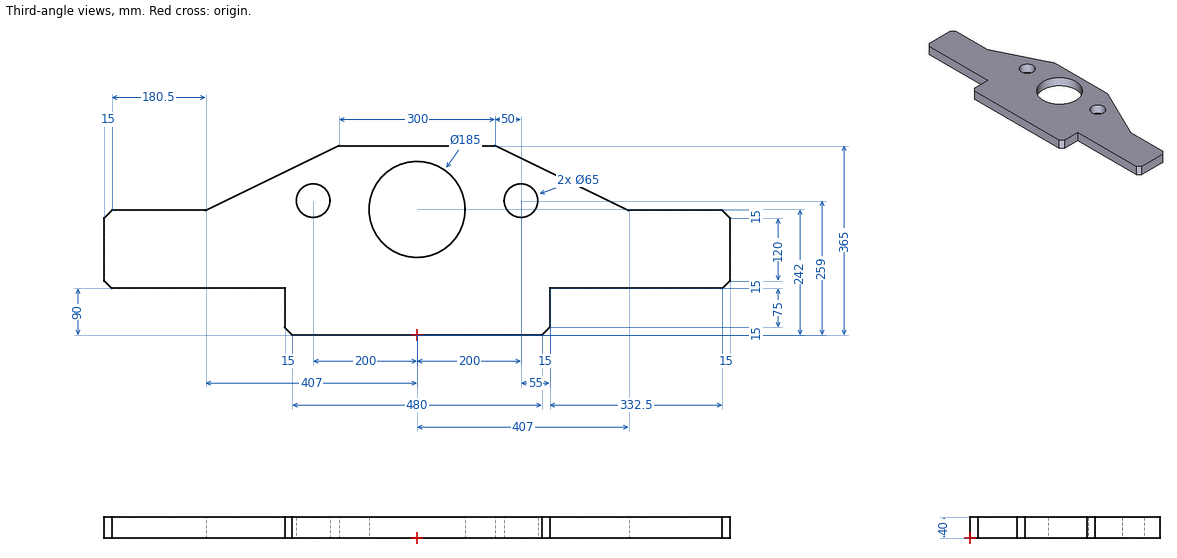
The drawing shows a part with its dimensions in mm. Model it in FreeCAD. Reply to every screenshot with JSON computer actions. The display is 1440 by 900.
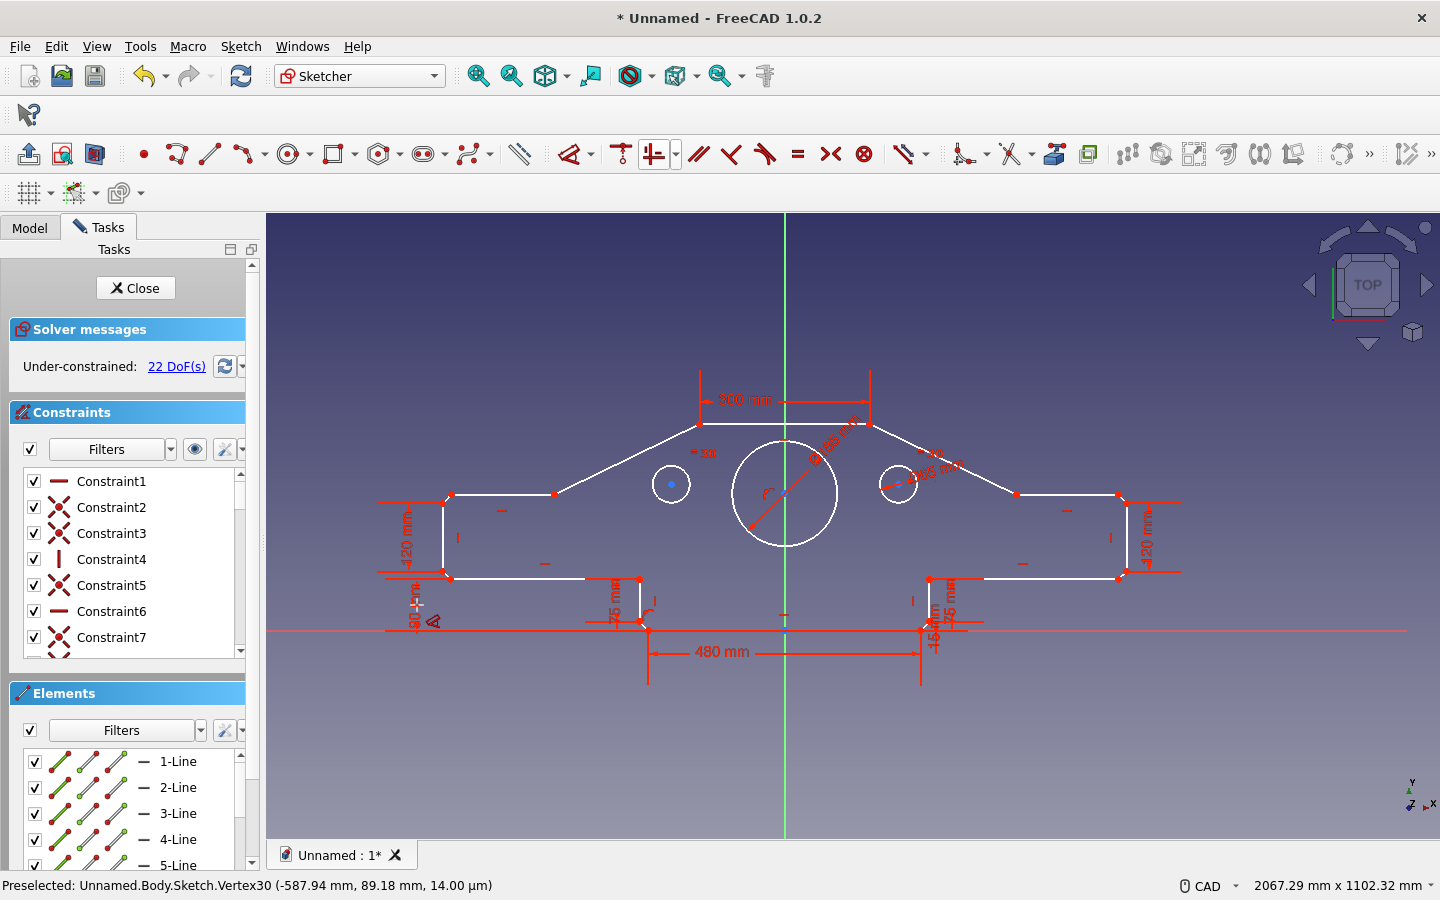
{"action": "scroll", "coordinate": [926, 625], "scroll_direction": "up", "scroll_amount": 8}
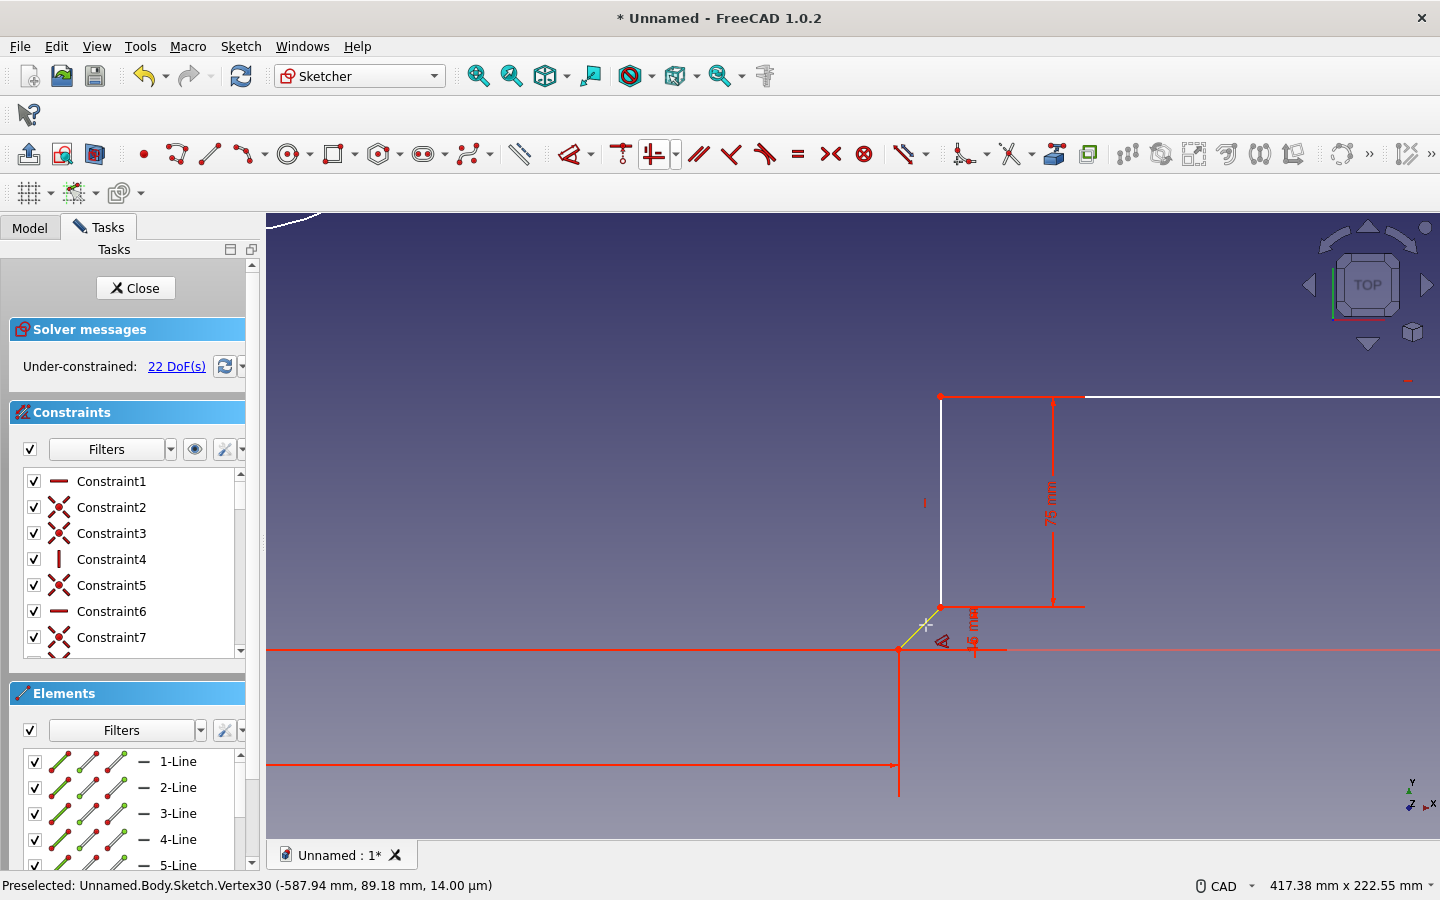
{"action": "left_click", "coordinate": [924, 624]}
{"action": "left_click", "coordinate": [920, 684]}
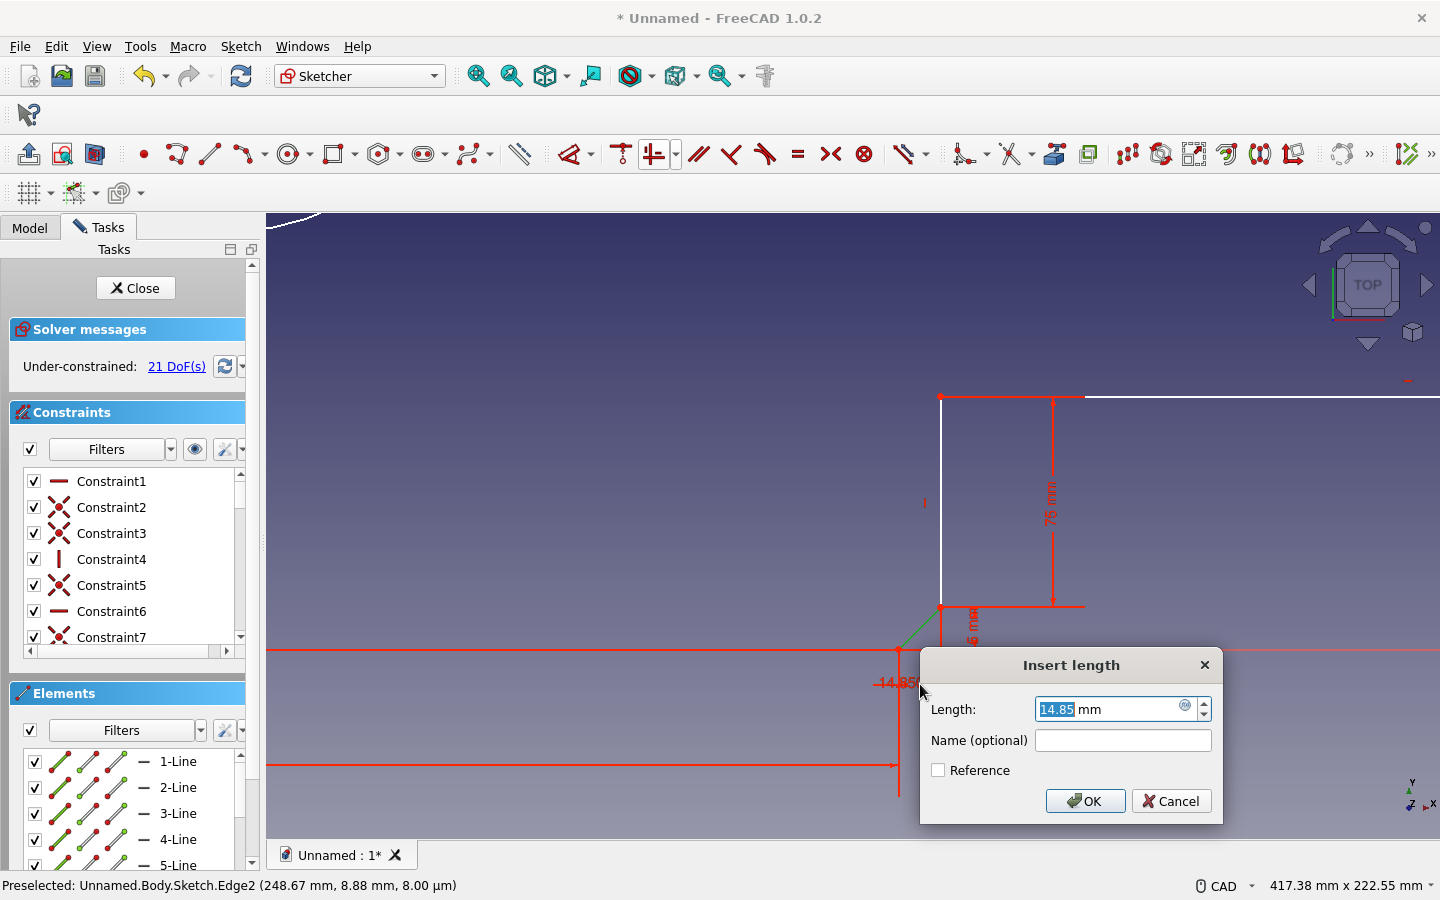
{"action": "type", "text": "15"}
{"action": "key", "text": "Return"}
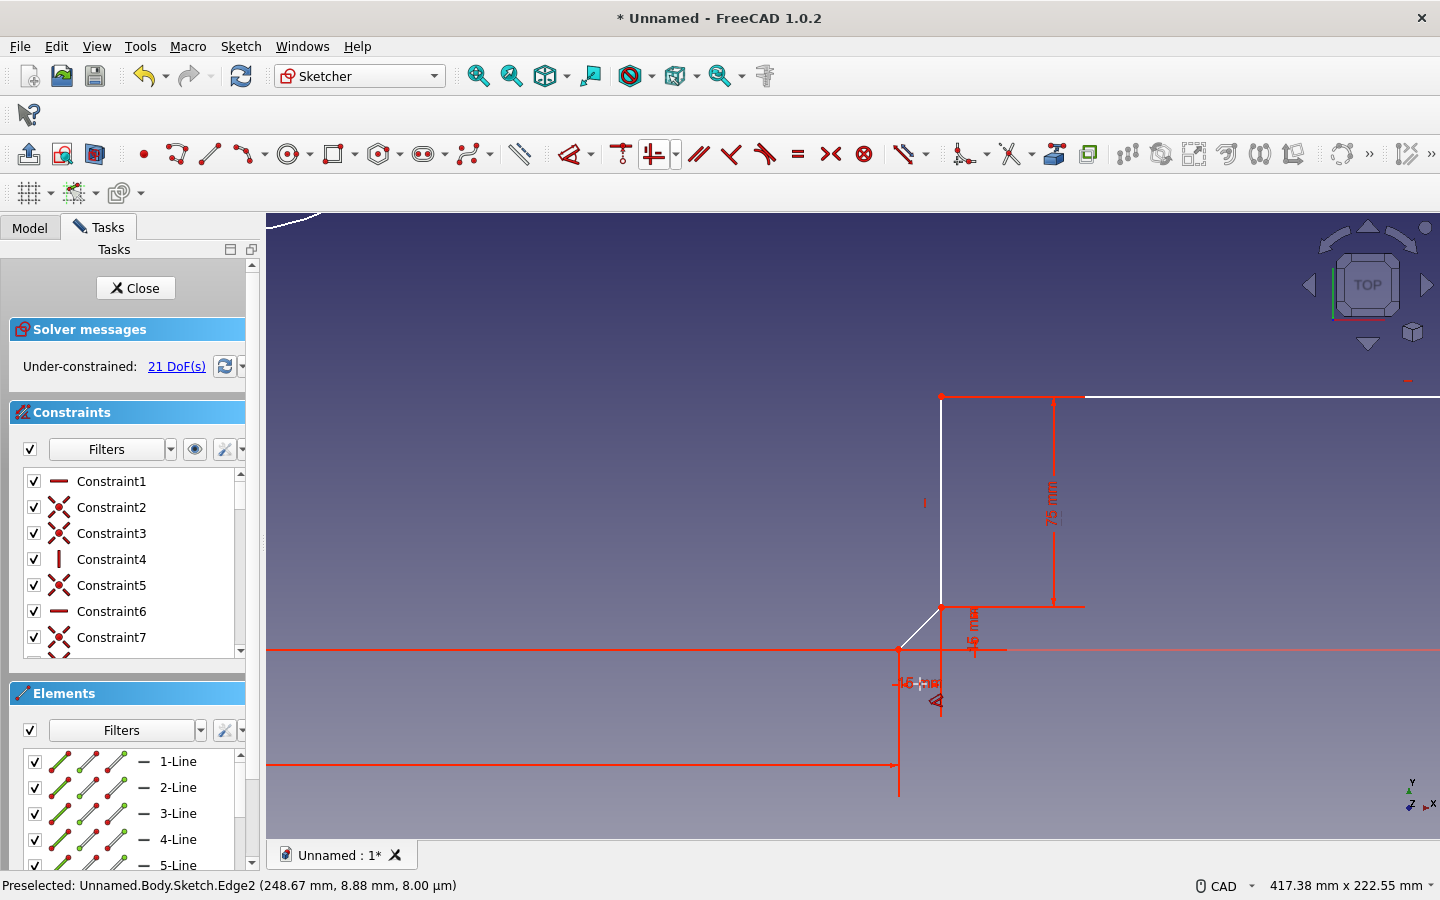
{"action": "scroll", "coordinate": [926, 625], "scroll_direction": "down", "scroll_amount": 8}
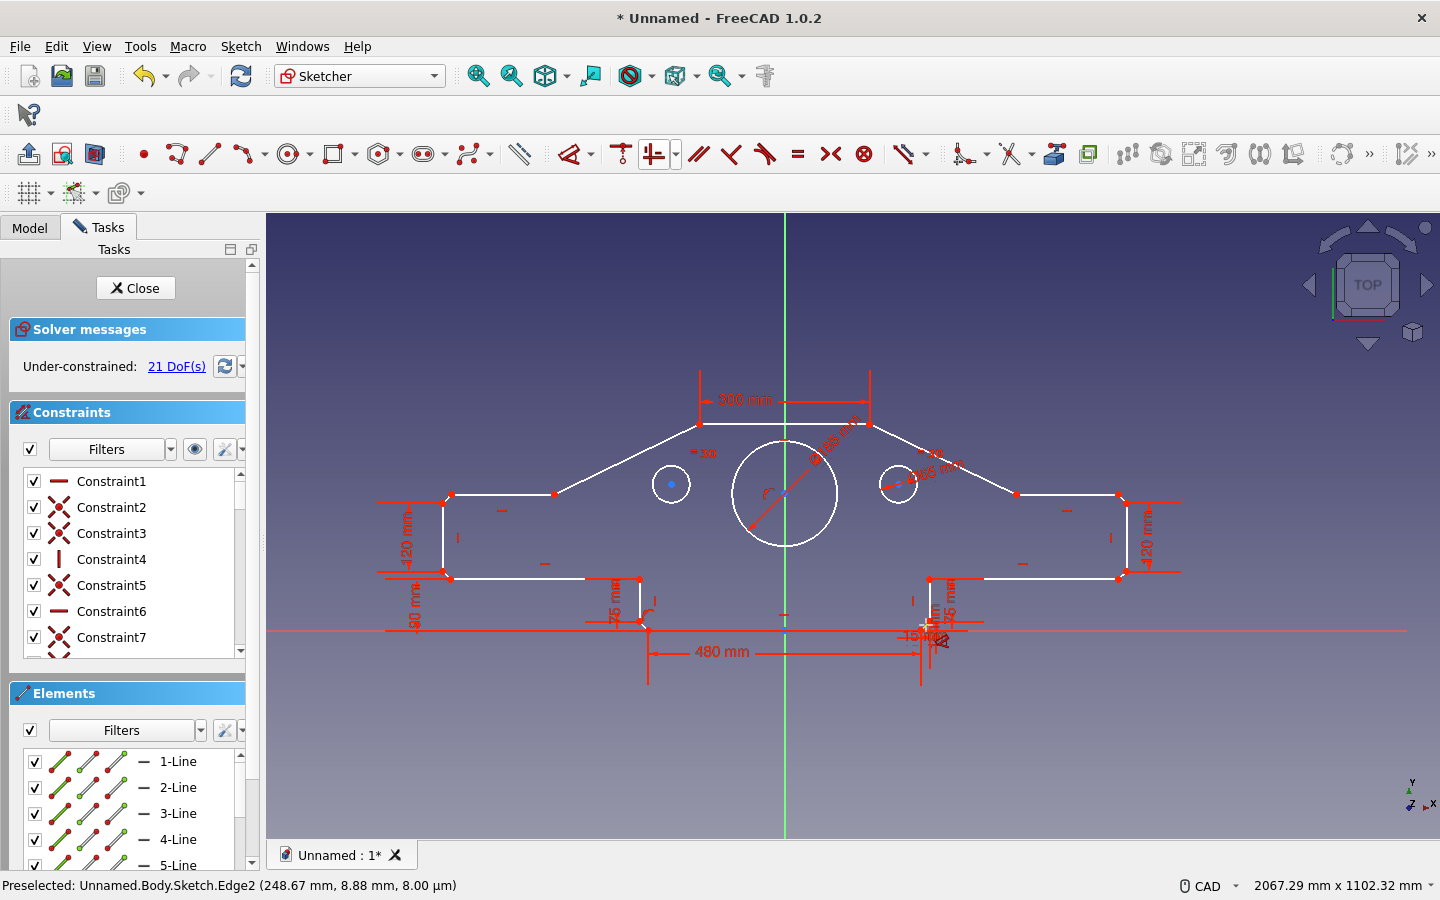
{"action": "scroll", "coordinate": [1121, 577], "scroll_direction": "up", "scroll_amount": 8}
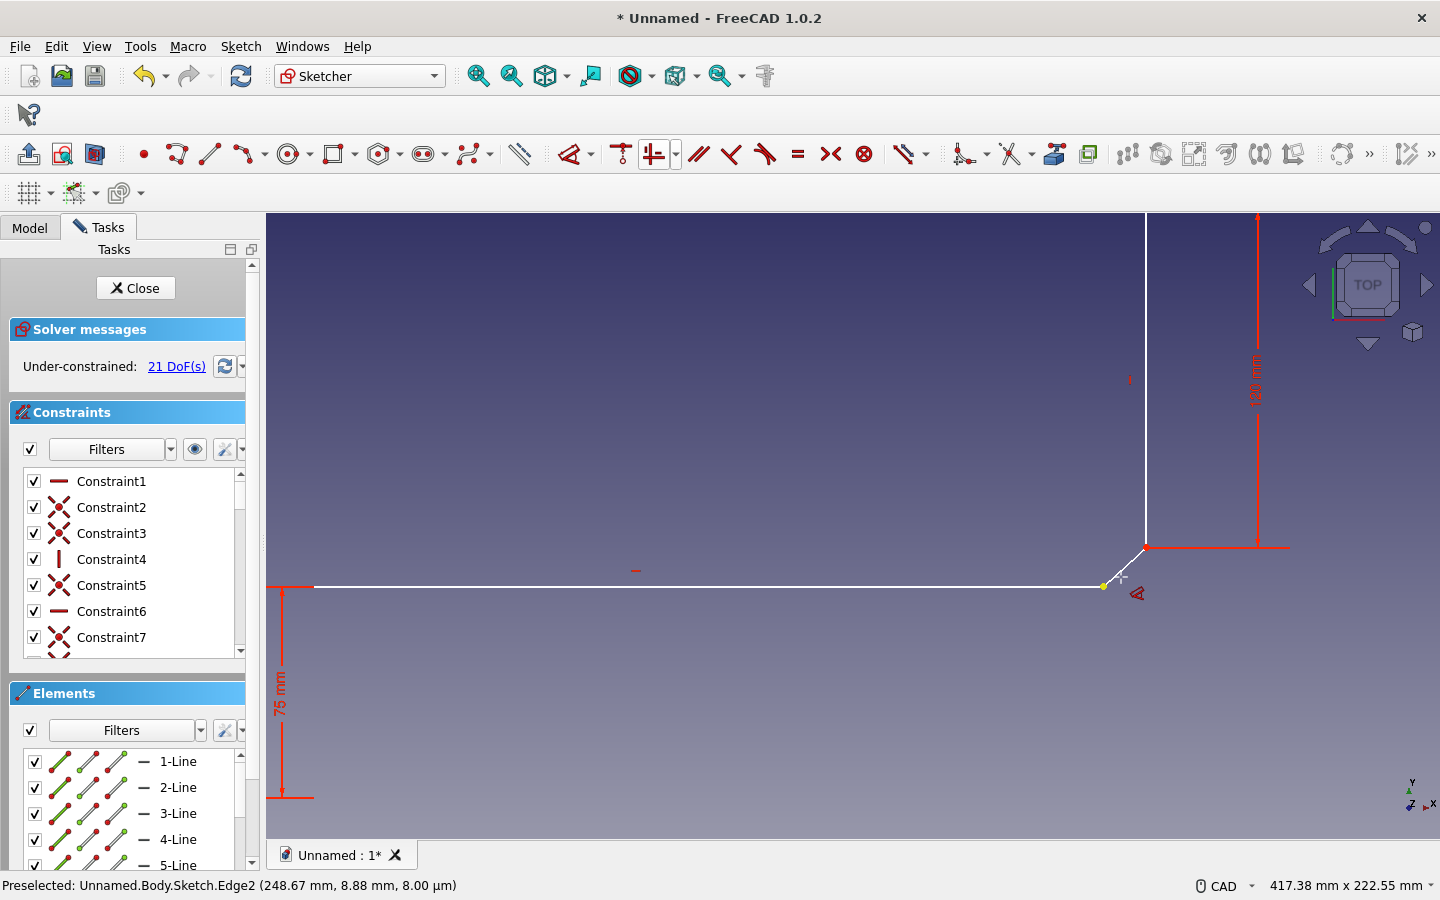
{"action": "left_click", "coordinate": [1117, 575]}
{"action": "left_click", "coordinate": [1125, 621]}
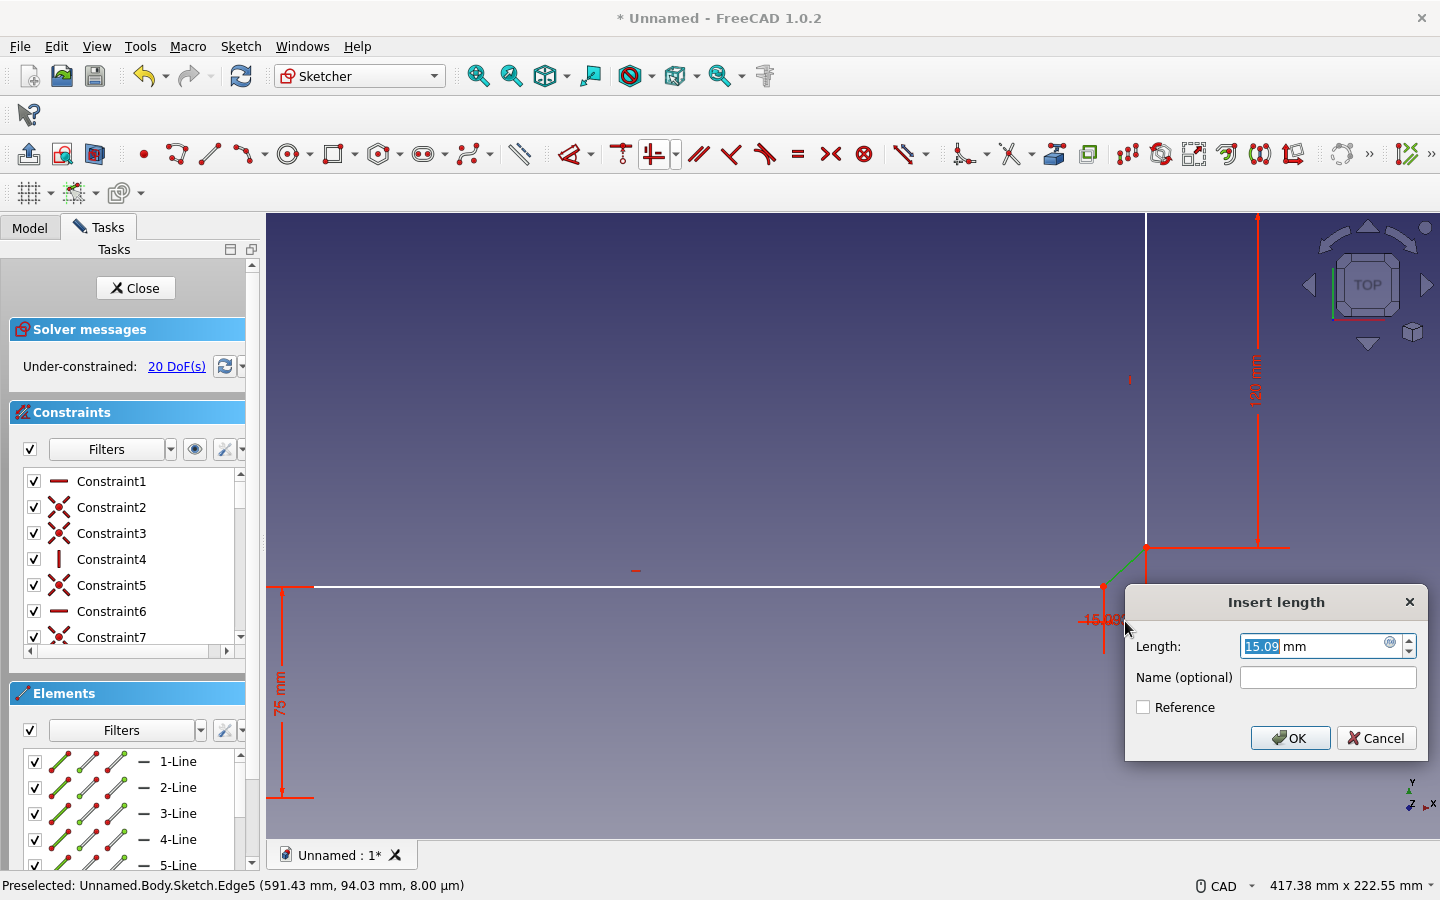
{"action": "type", "text": "15"}
{"action": "key", "text": "Return"}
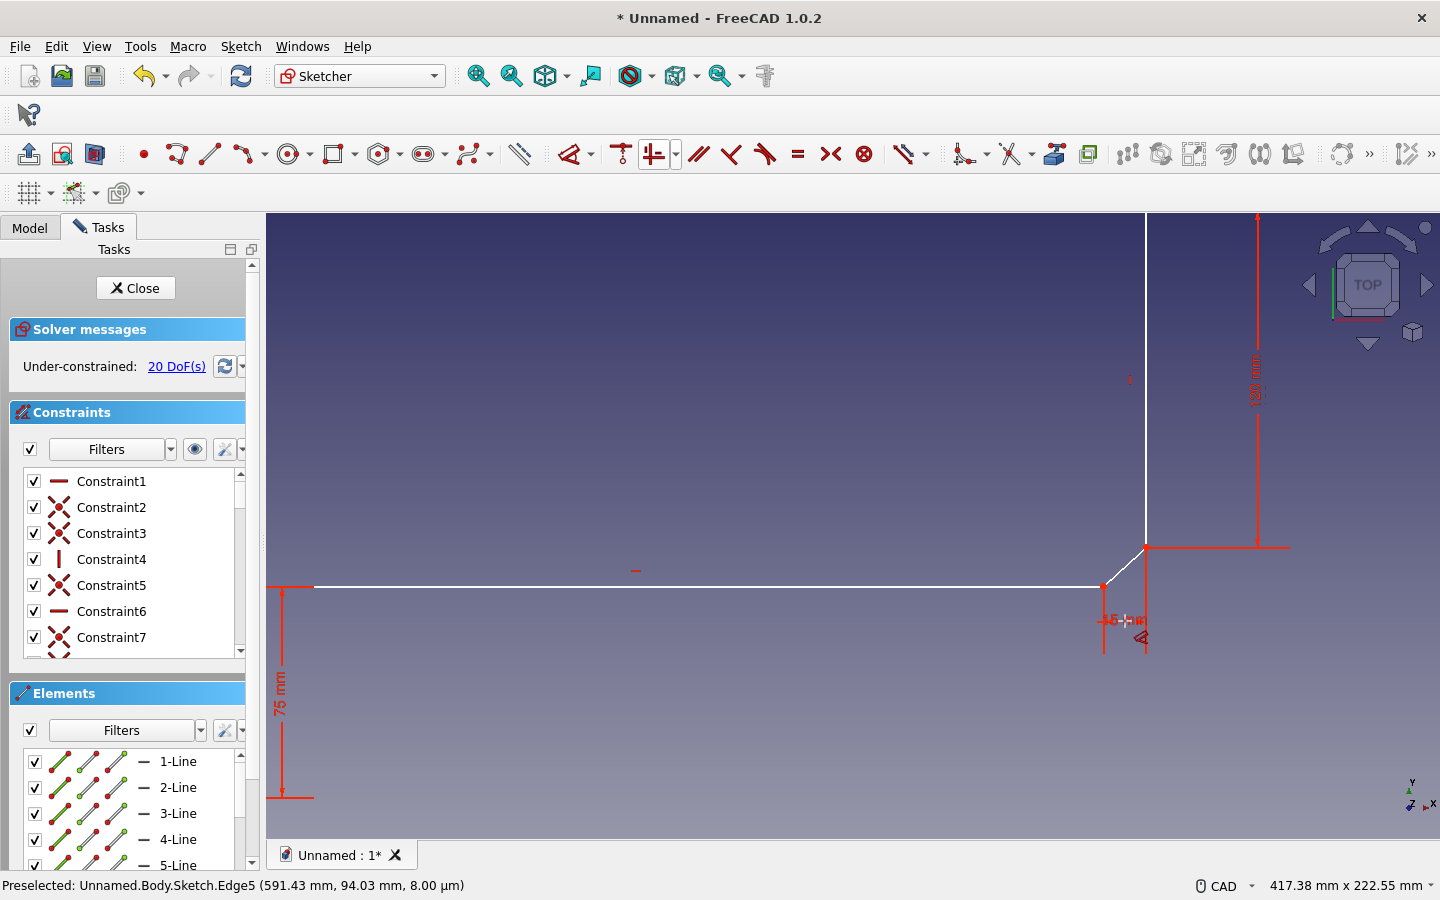
{"action": "left_click", "coordinate": [1116, 575]}
{"action": "left_click", "coordinate": [1180, 567]}